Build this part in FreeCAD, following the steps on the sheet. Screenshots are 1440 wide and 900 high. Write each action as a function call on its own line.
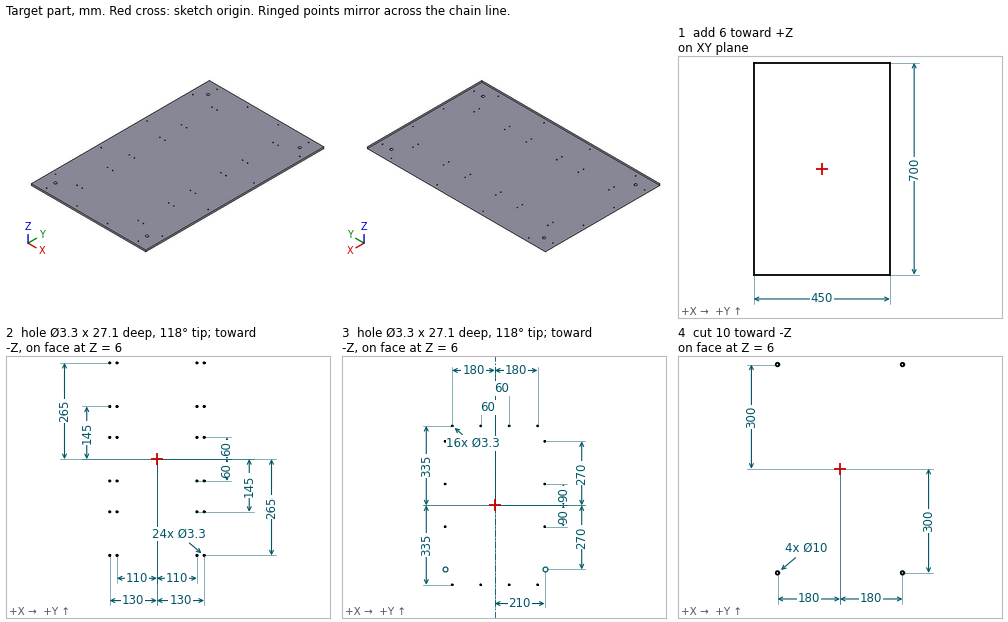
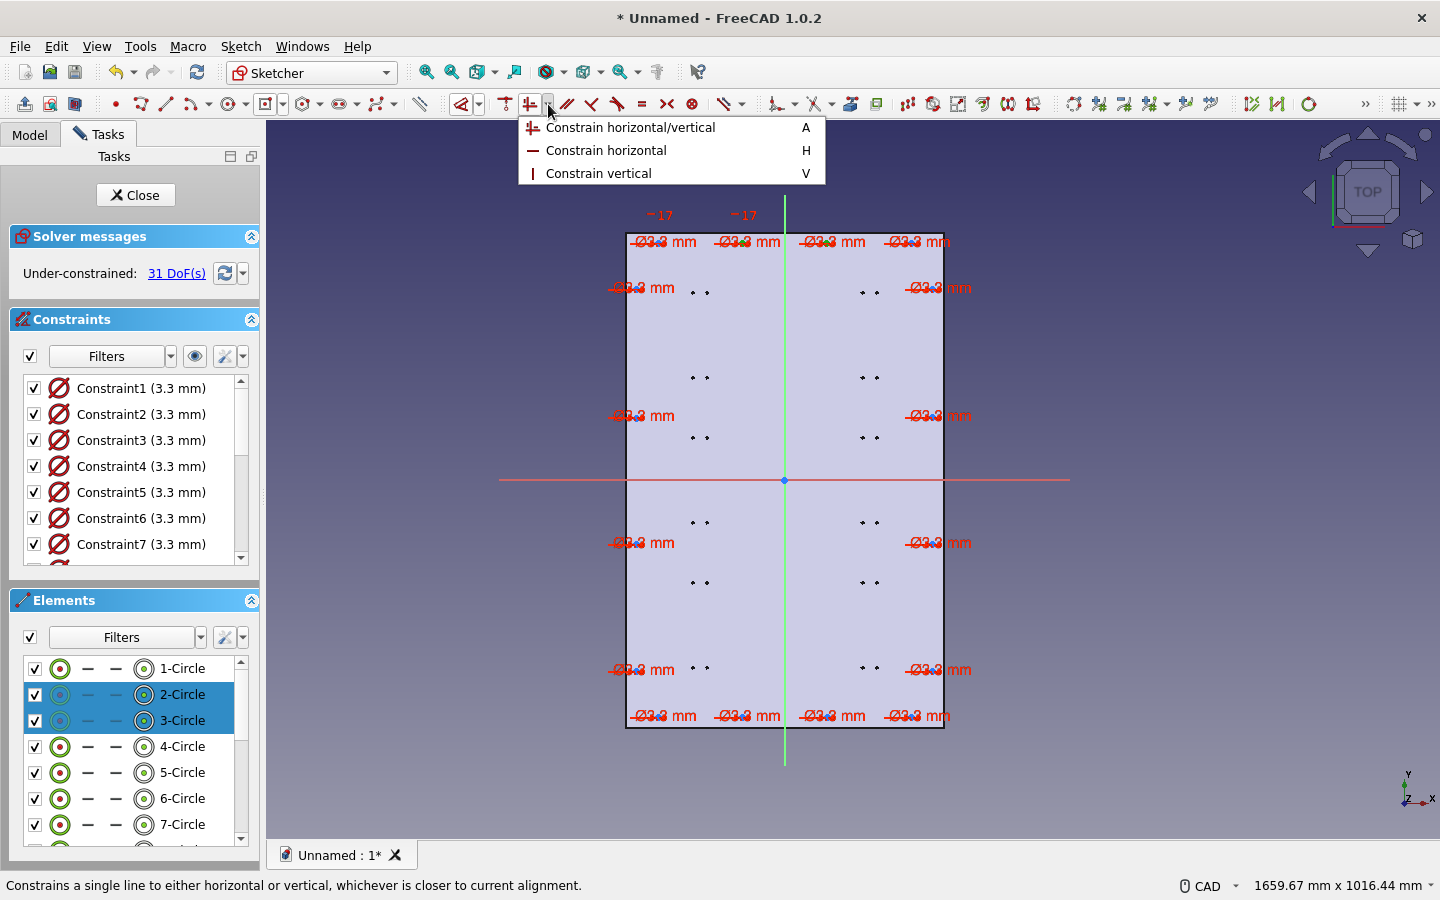
click(672, 150)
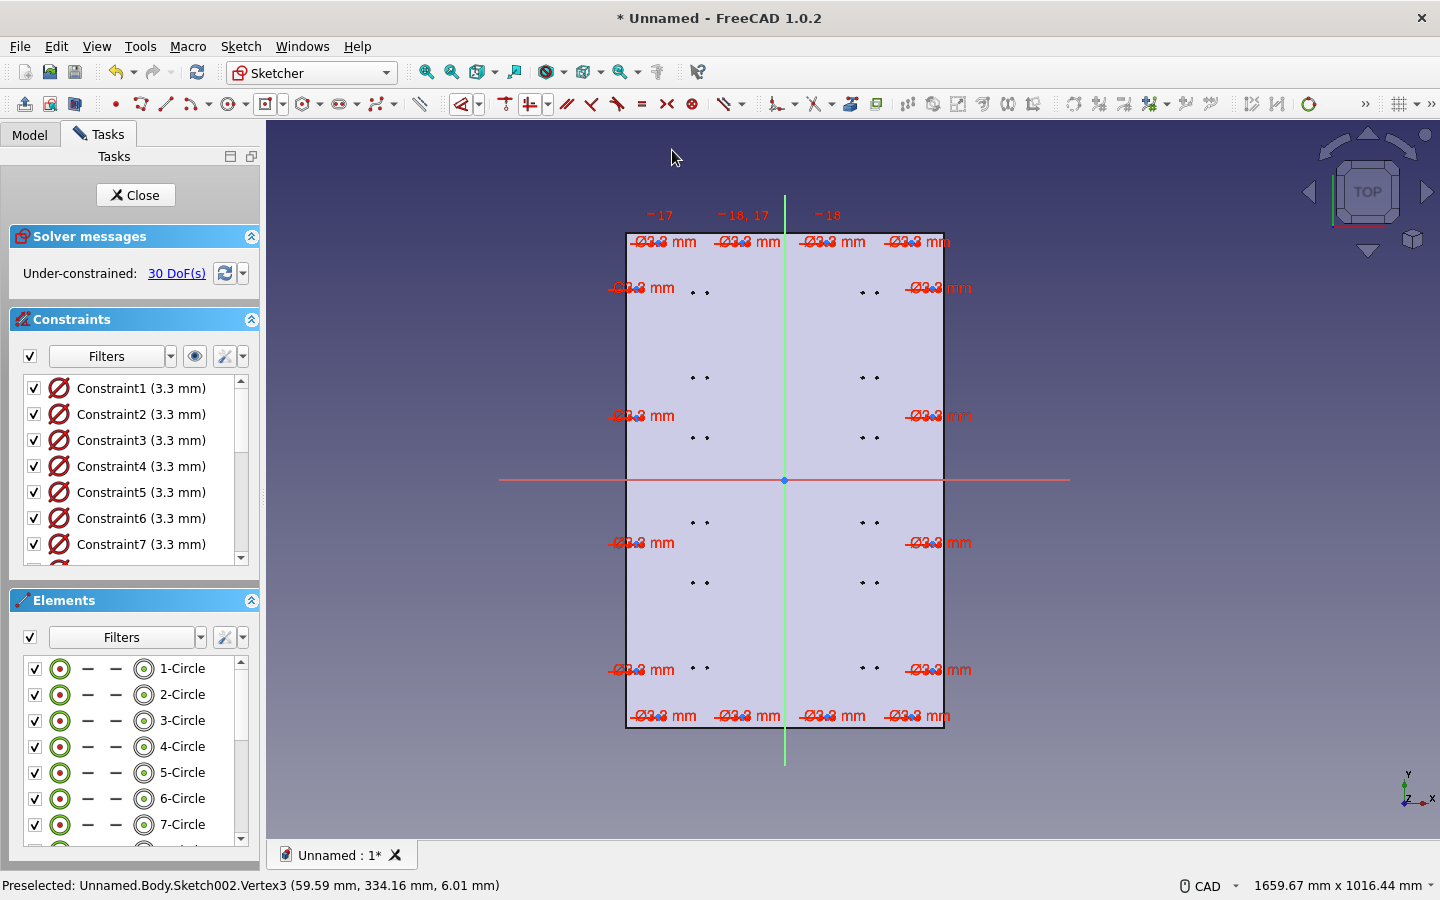
click(827, 244)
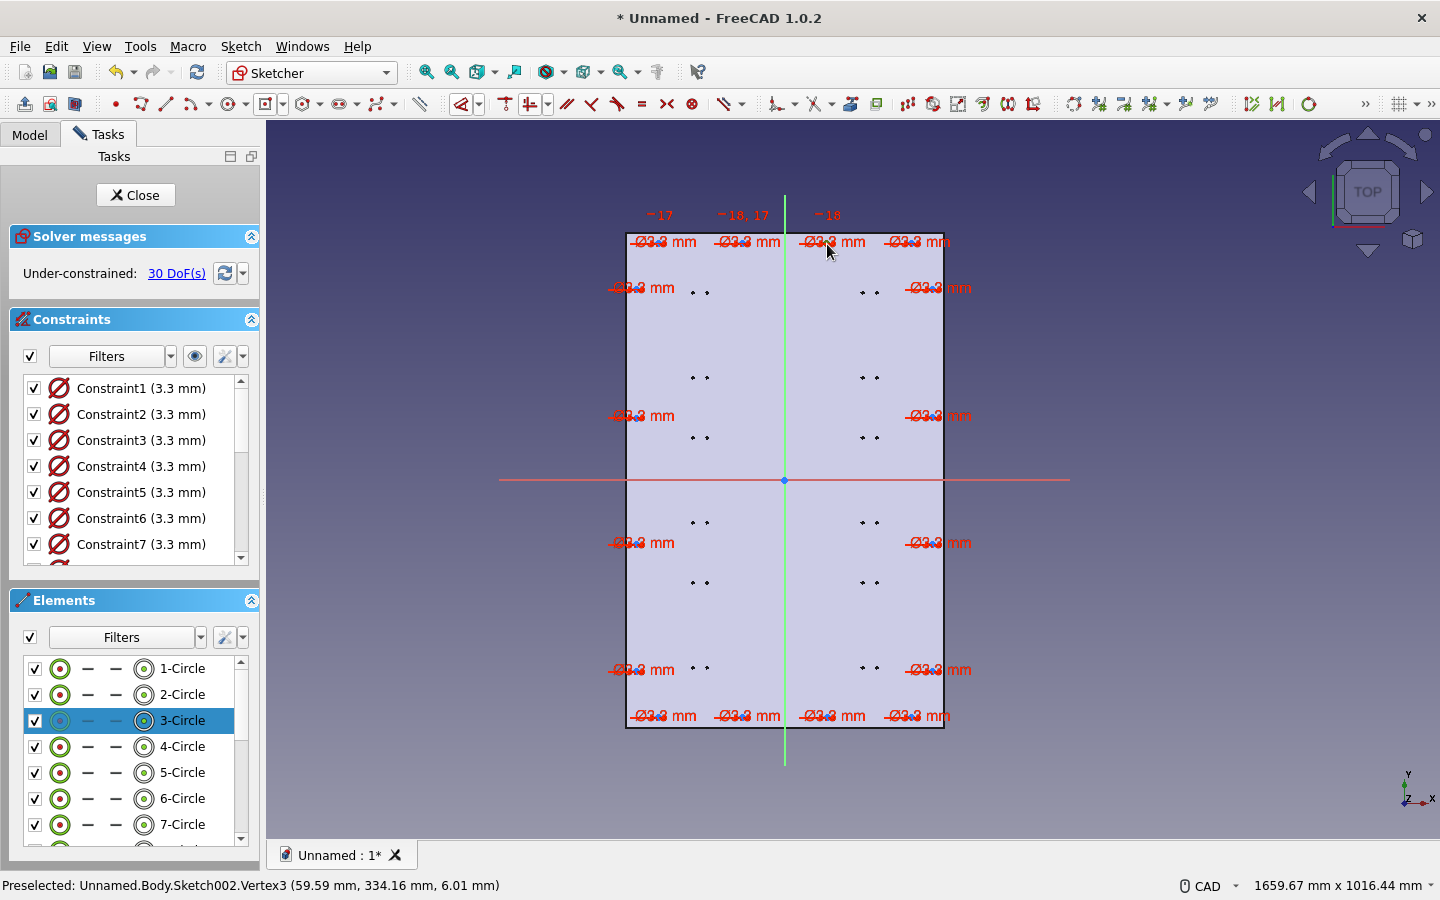
click(912, 244)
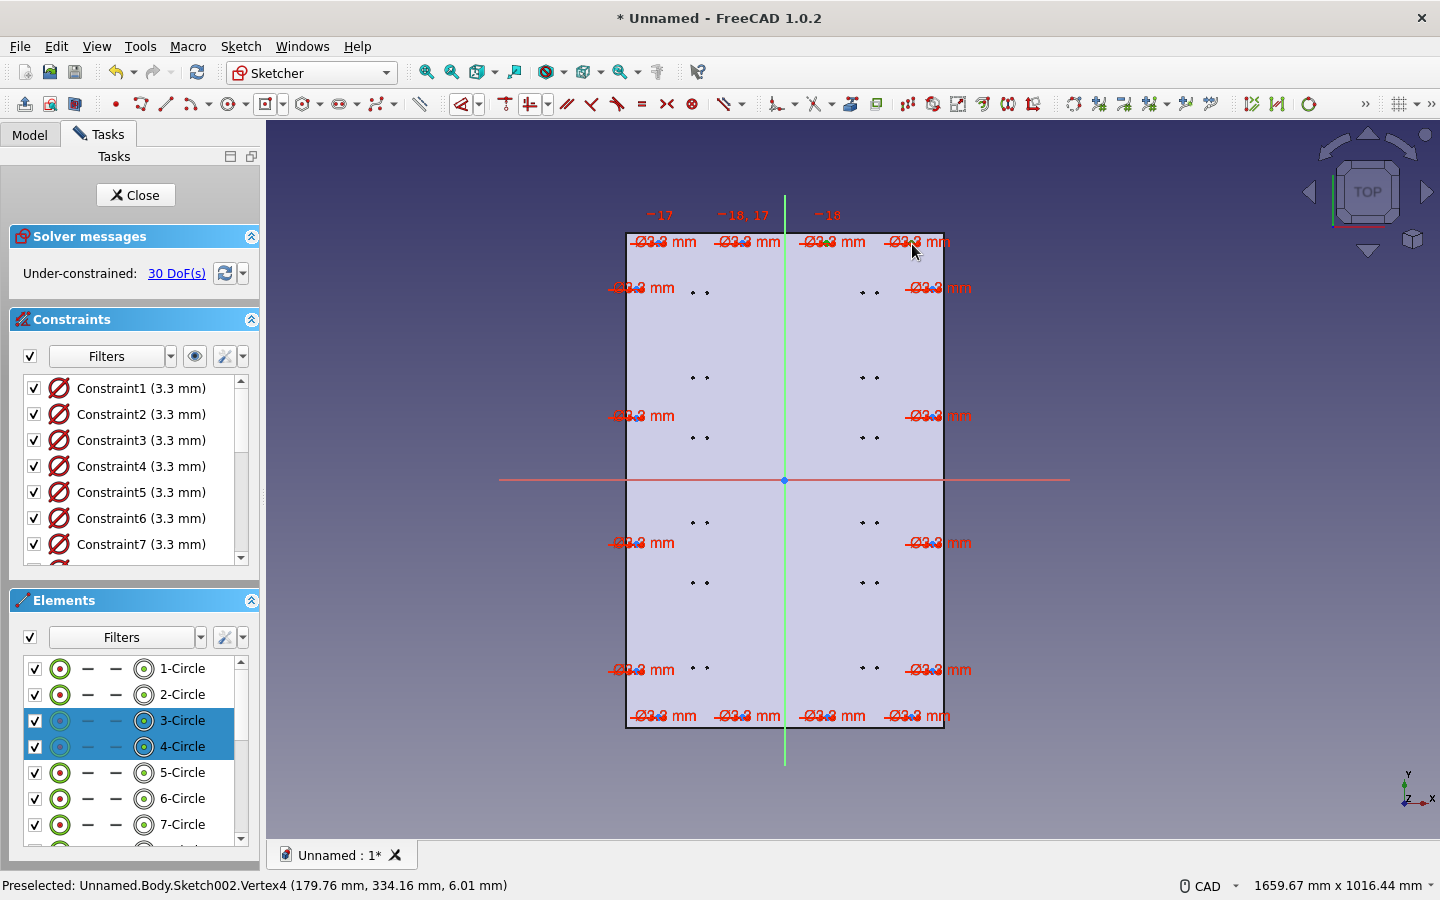
click(548, 104)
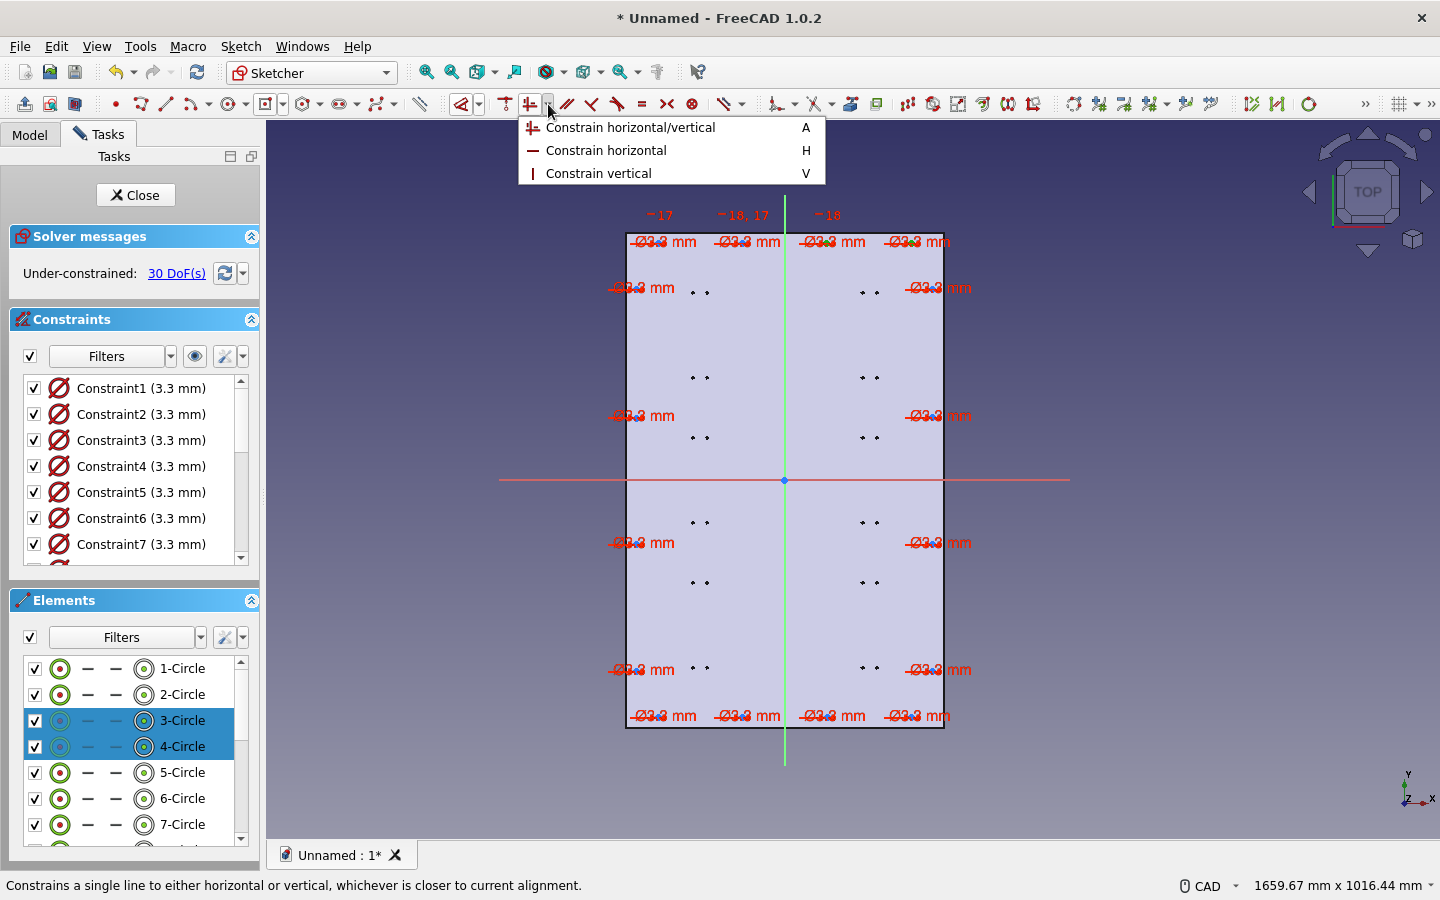
click(672, 150)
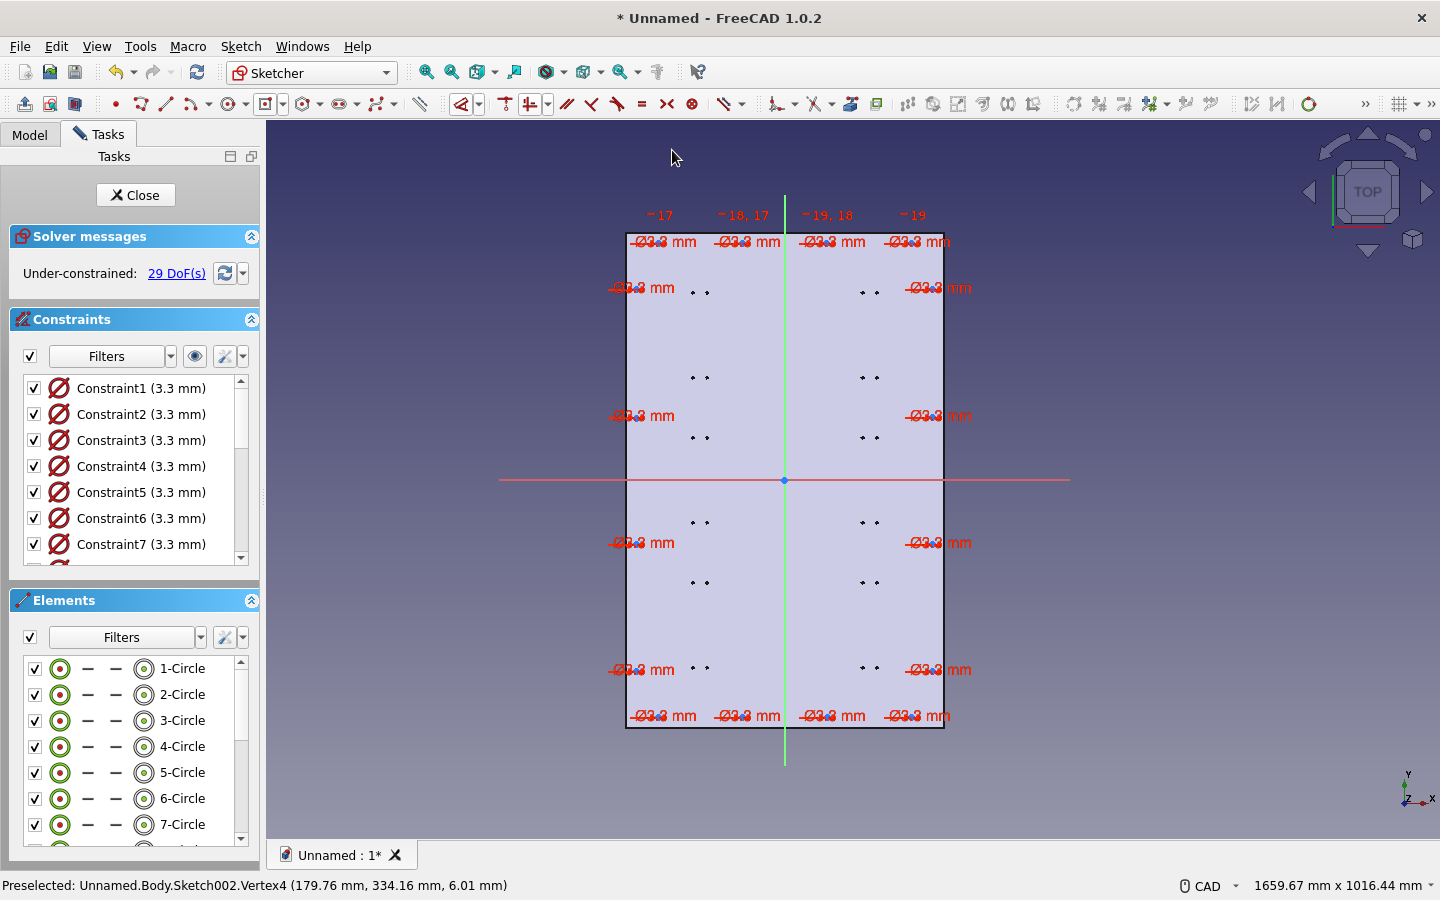
click(658, 244)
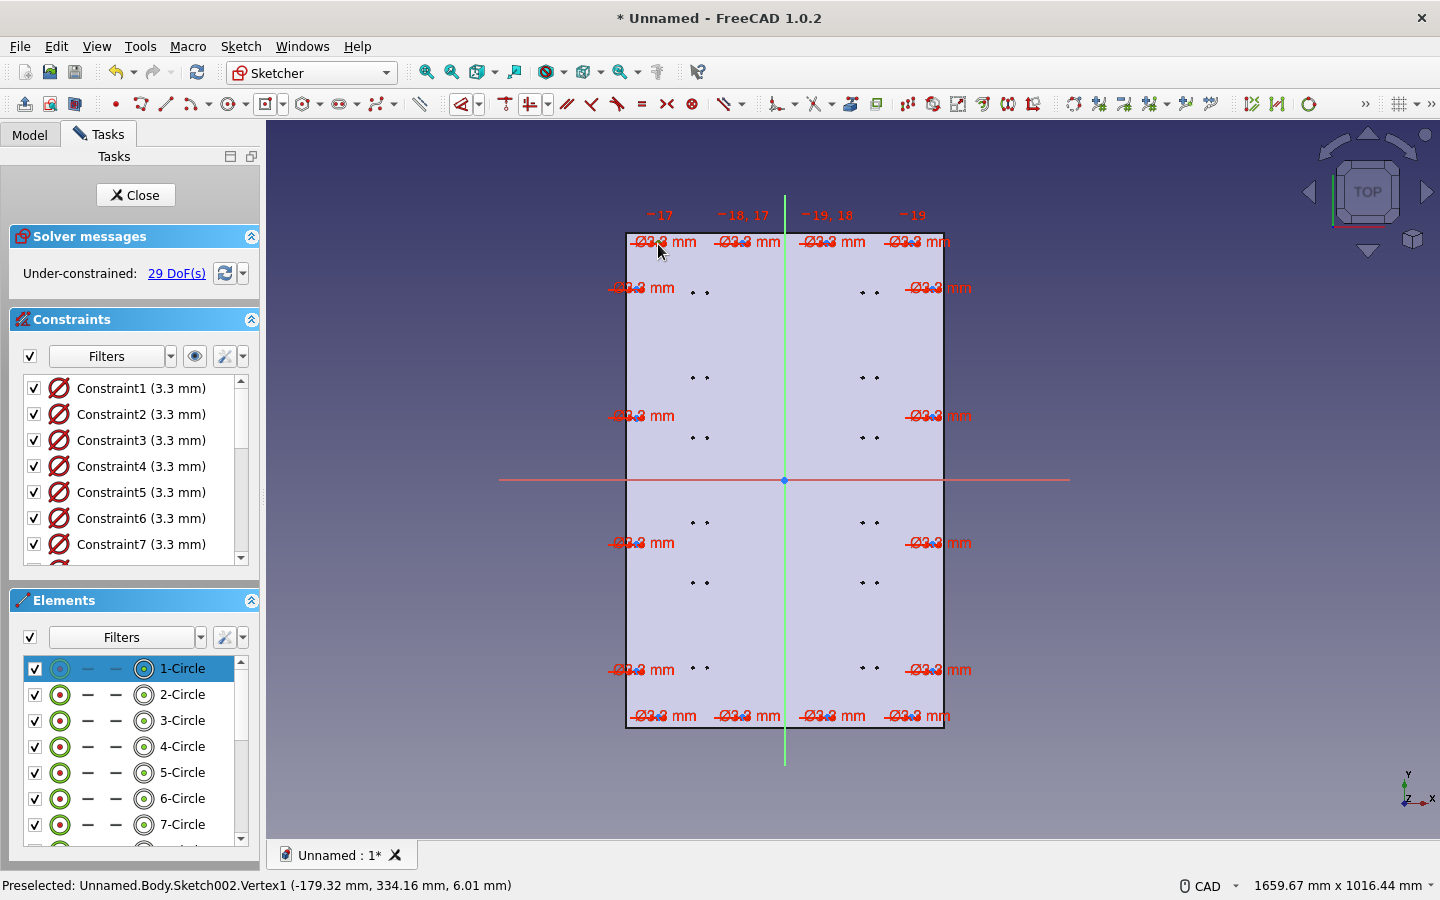
click(658, 718)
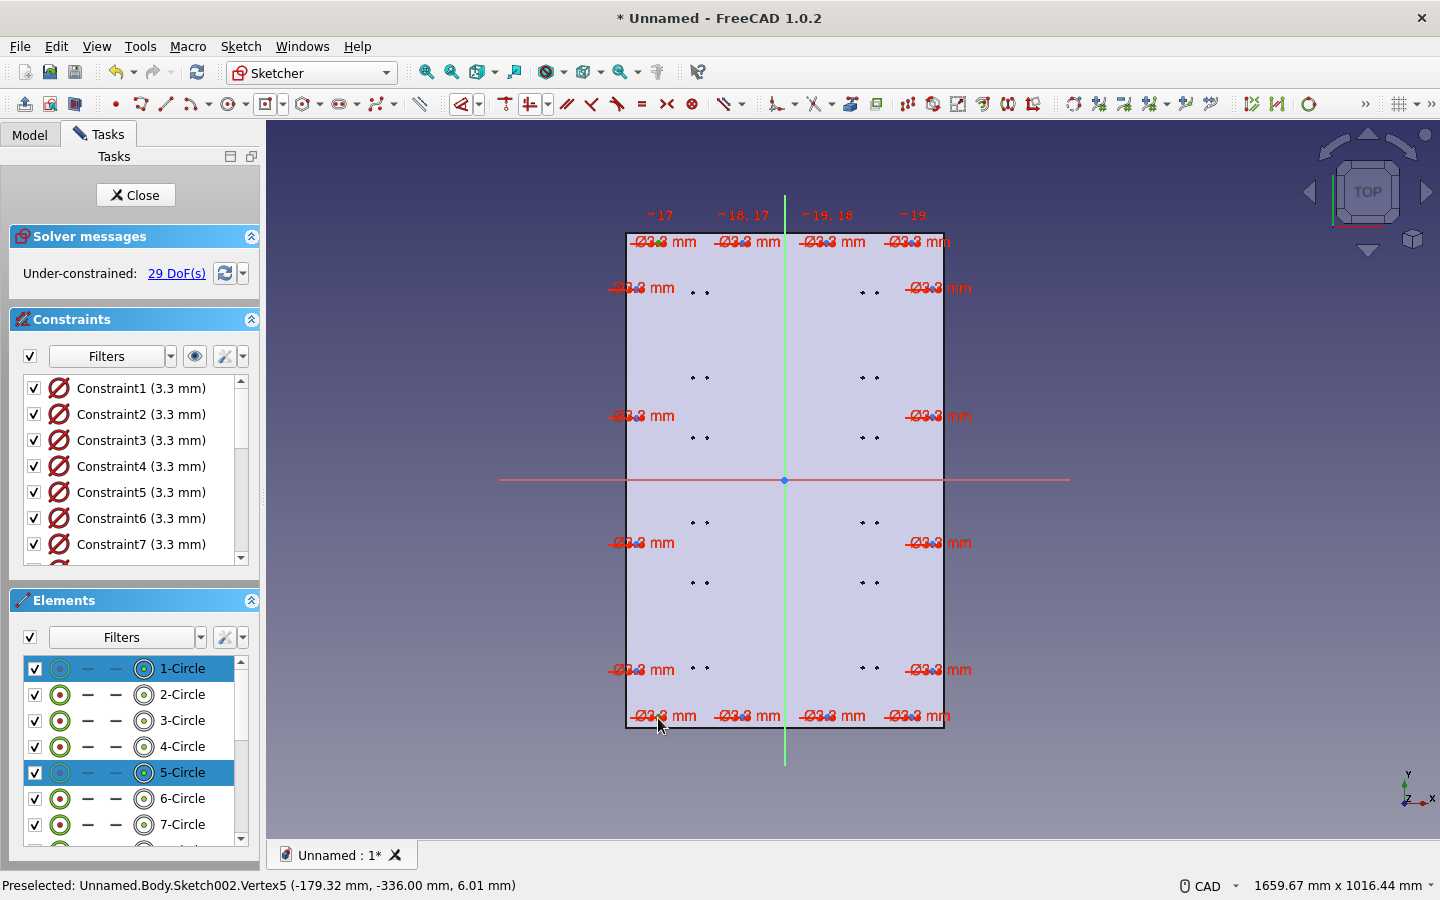
click(548, 104)